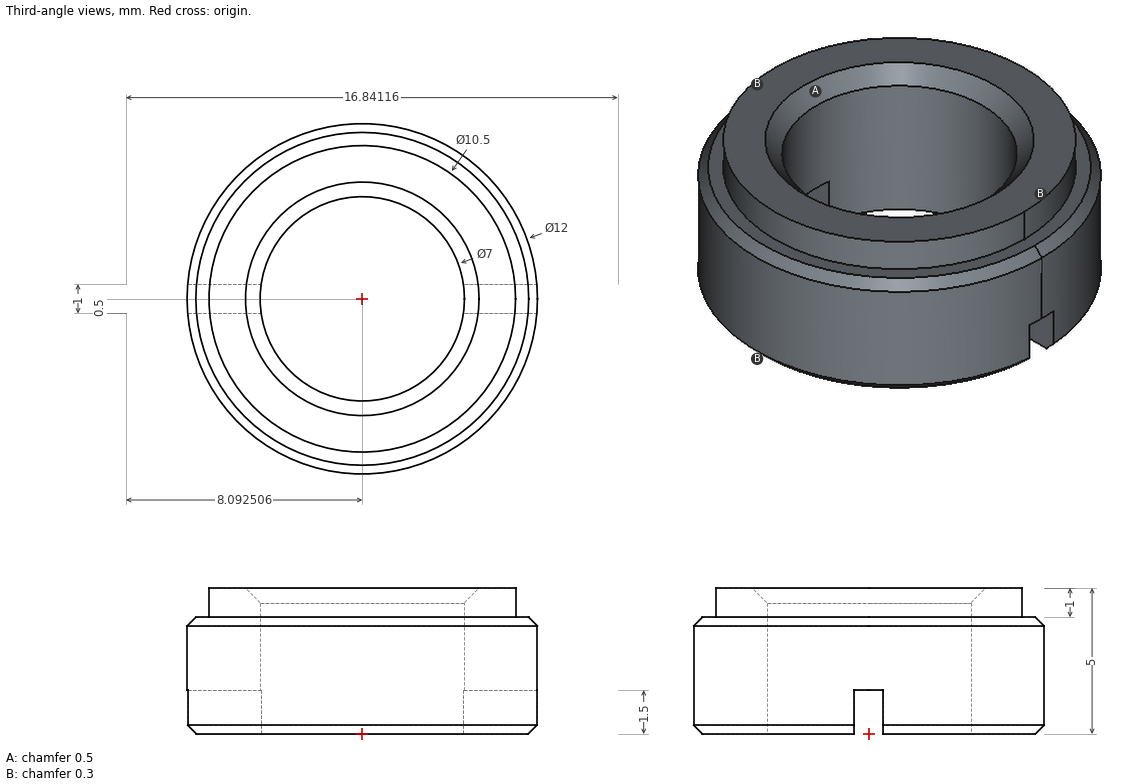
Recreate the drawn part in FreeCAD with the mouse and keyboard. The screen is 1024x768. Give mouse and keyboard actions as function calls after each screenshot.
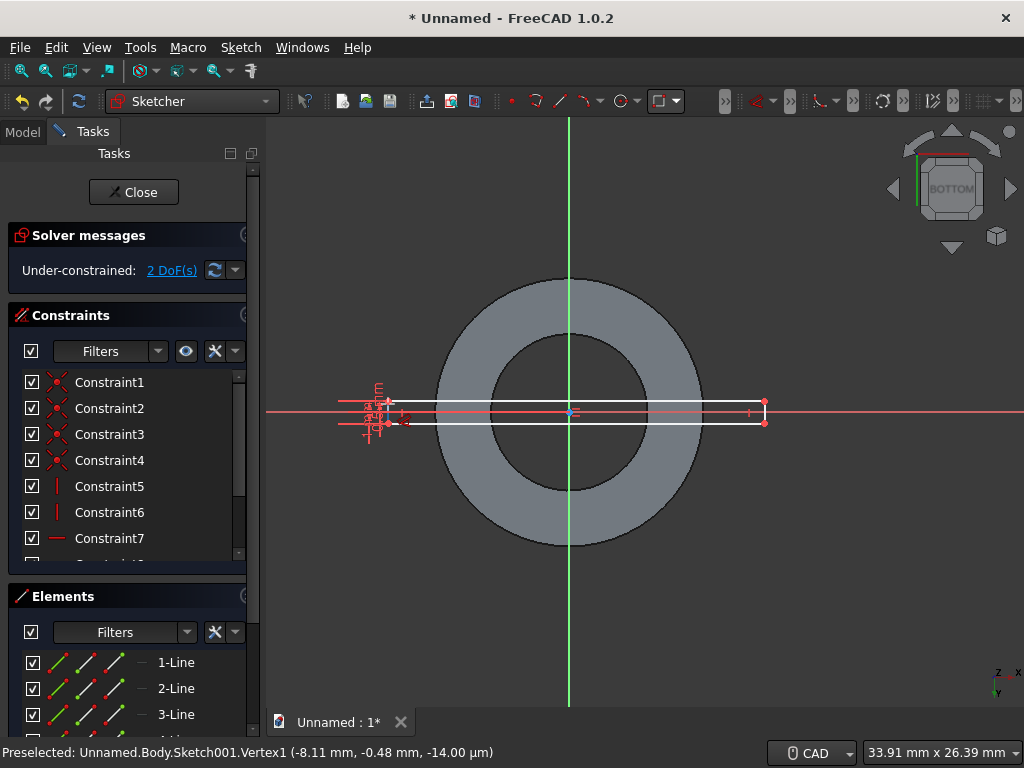
scroll(501, 424, up, 2)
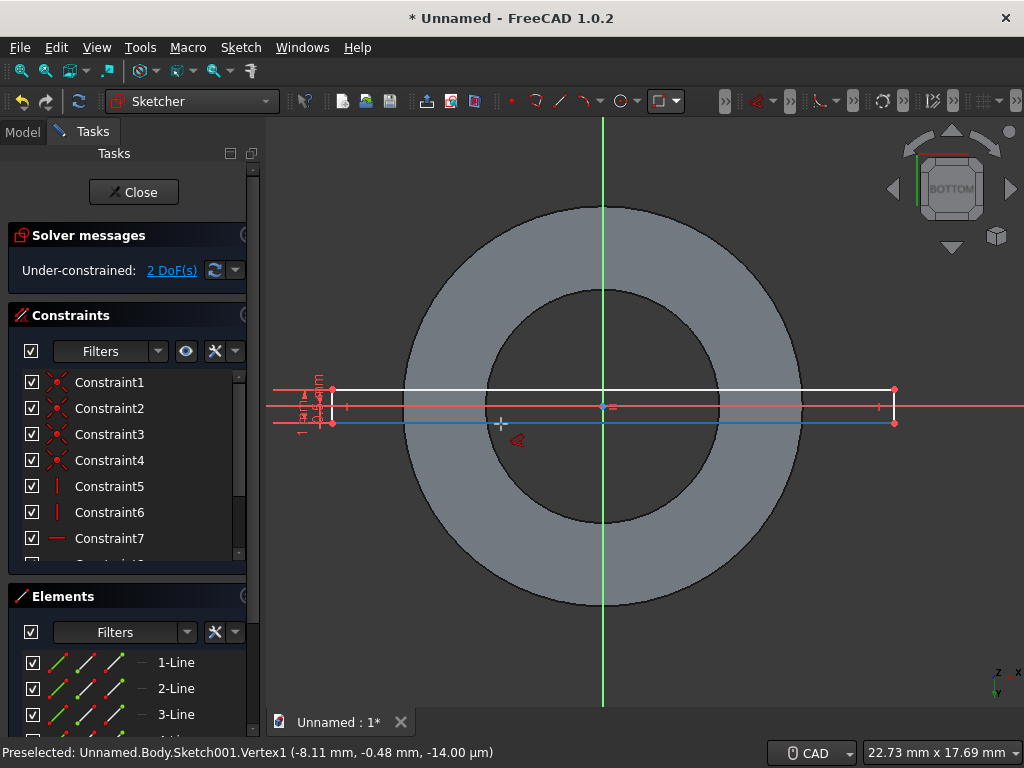
click(501, 423)
click(475, 457)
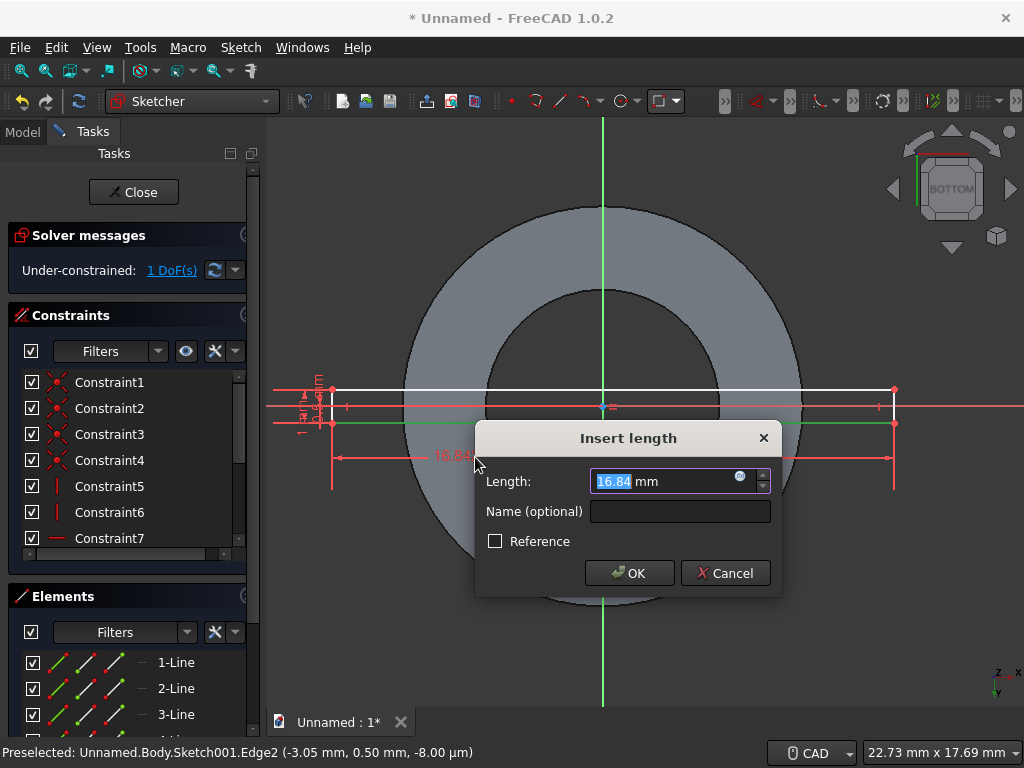
text(16.84116)
key(Return)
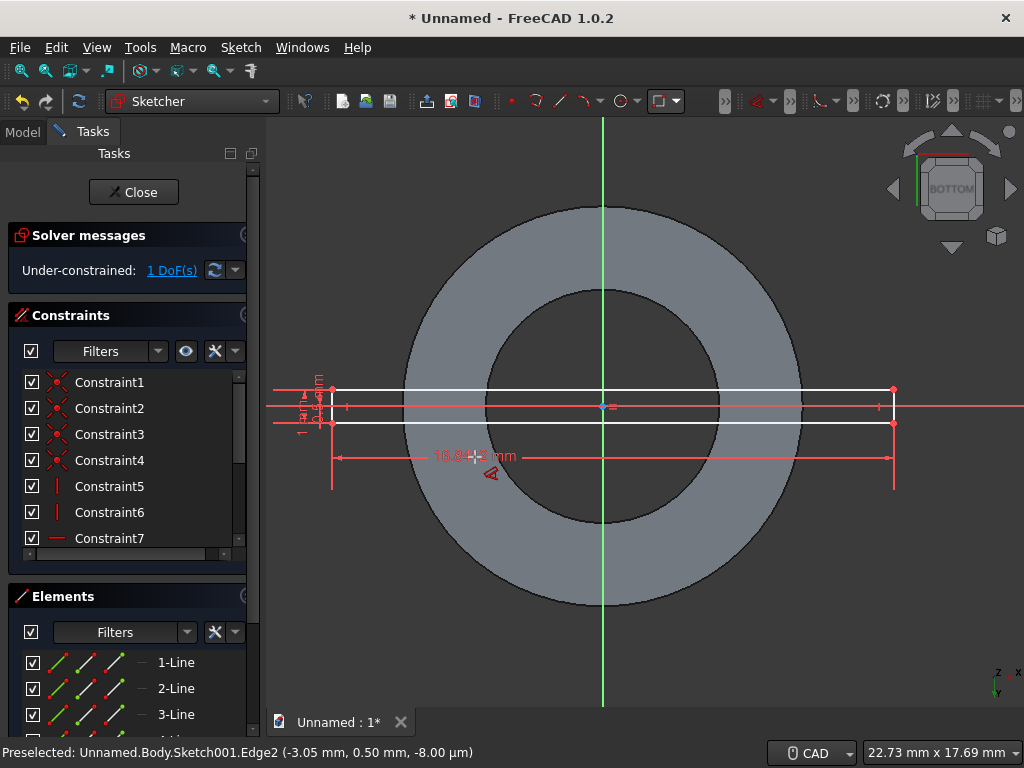
click(332, 390)
click(467, 356)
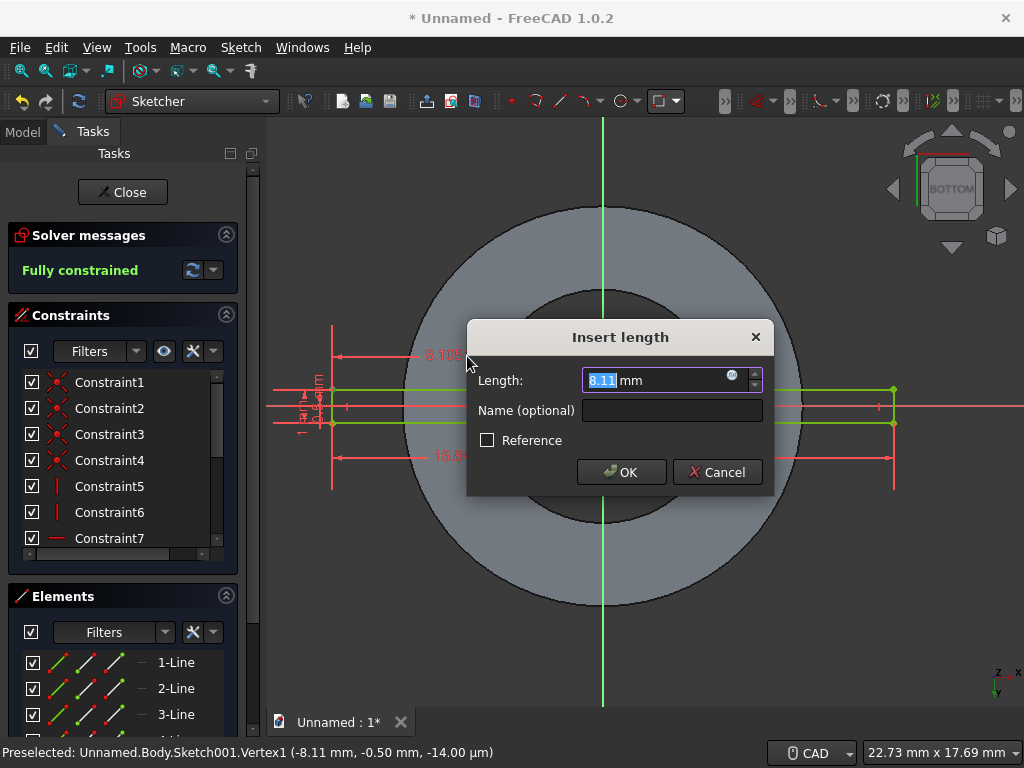
text(8.092506)
key(Return)
key(Escape)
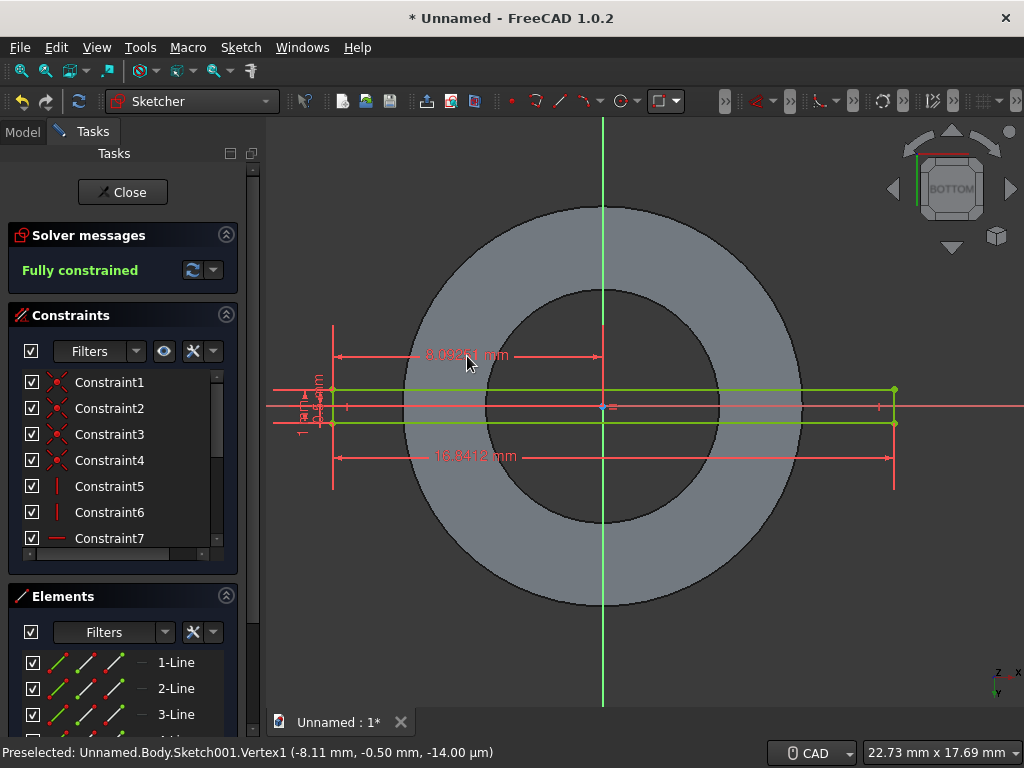
click(123, 192)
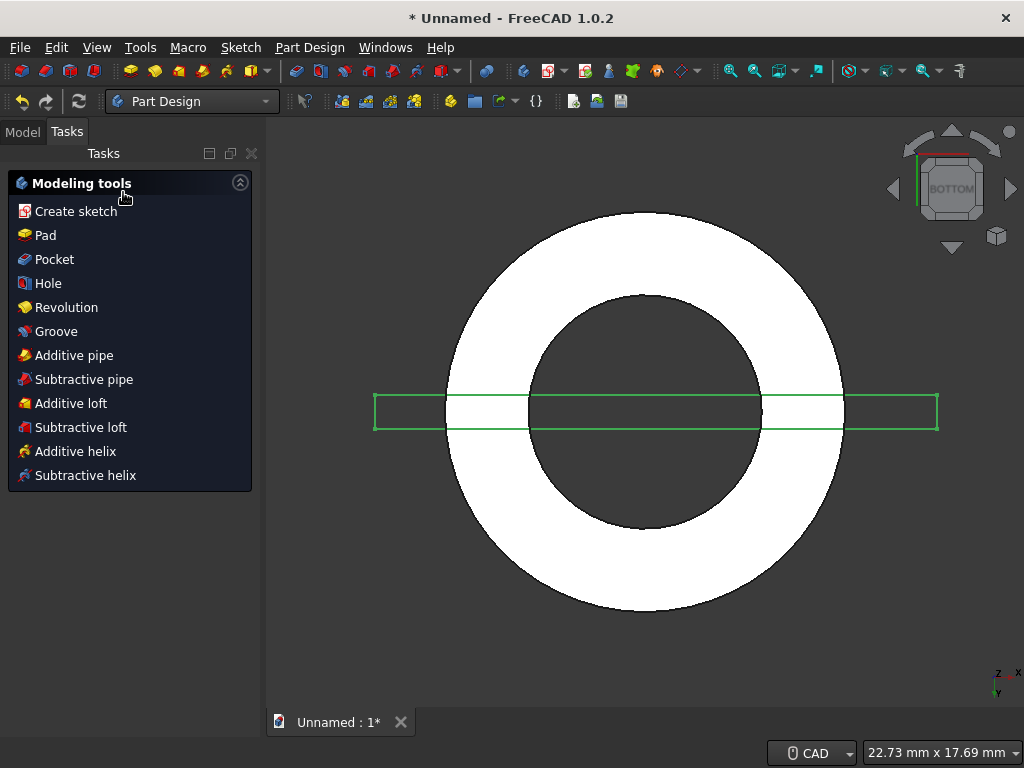
click(298, 72)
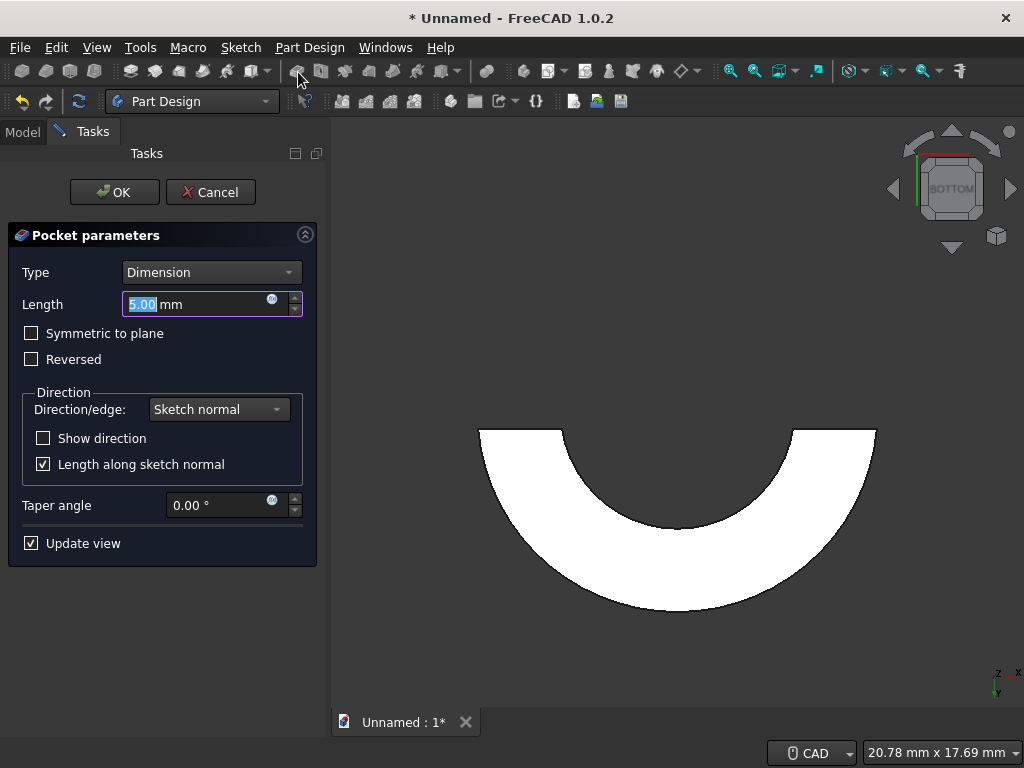
text(1.5)
key(Tab)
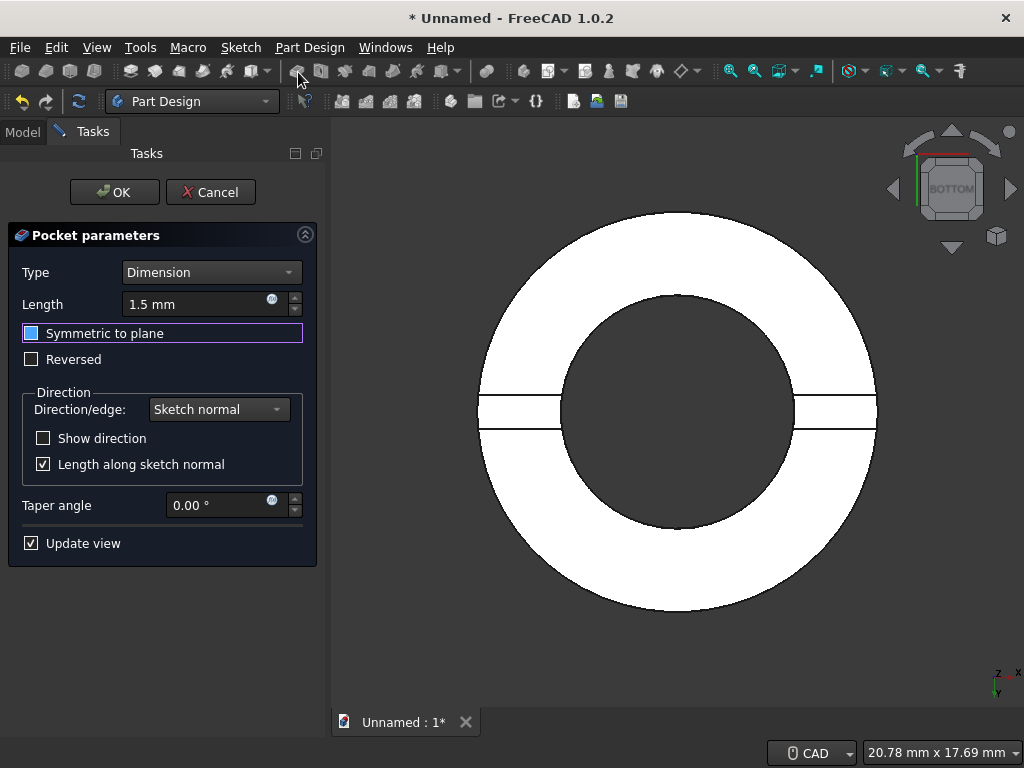
click(115, 192)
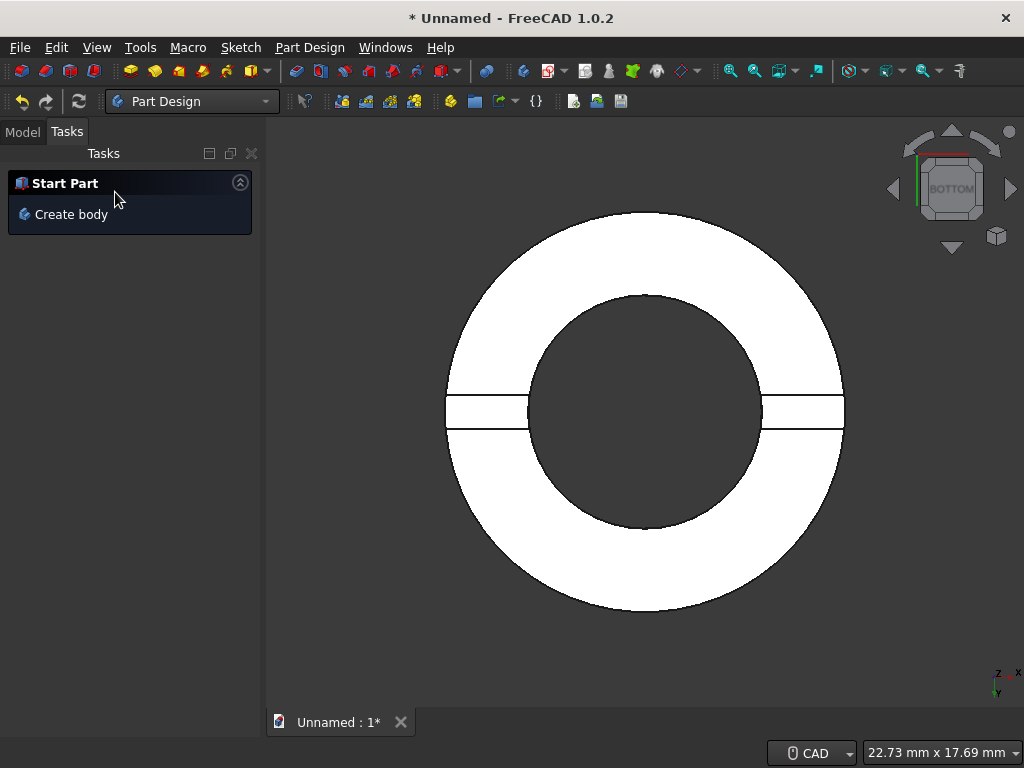
click(23, 131)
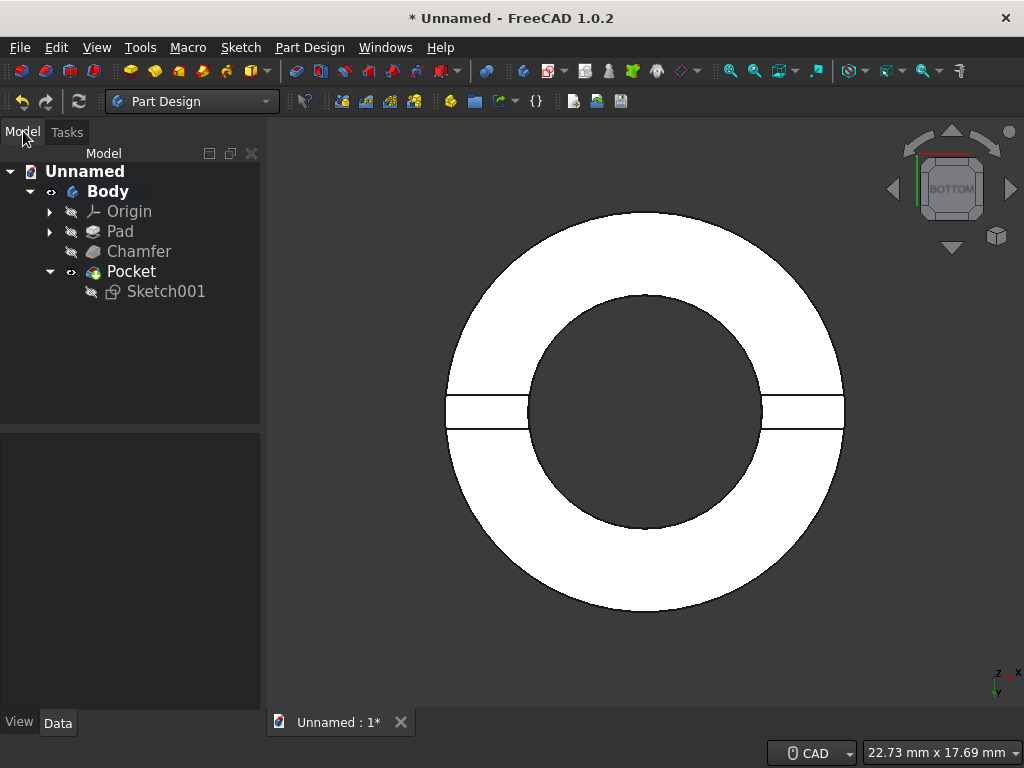
click(50, 212)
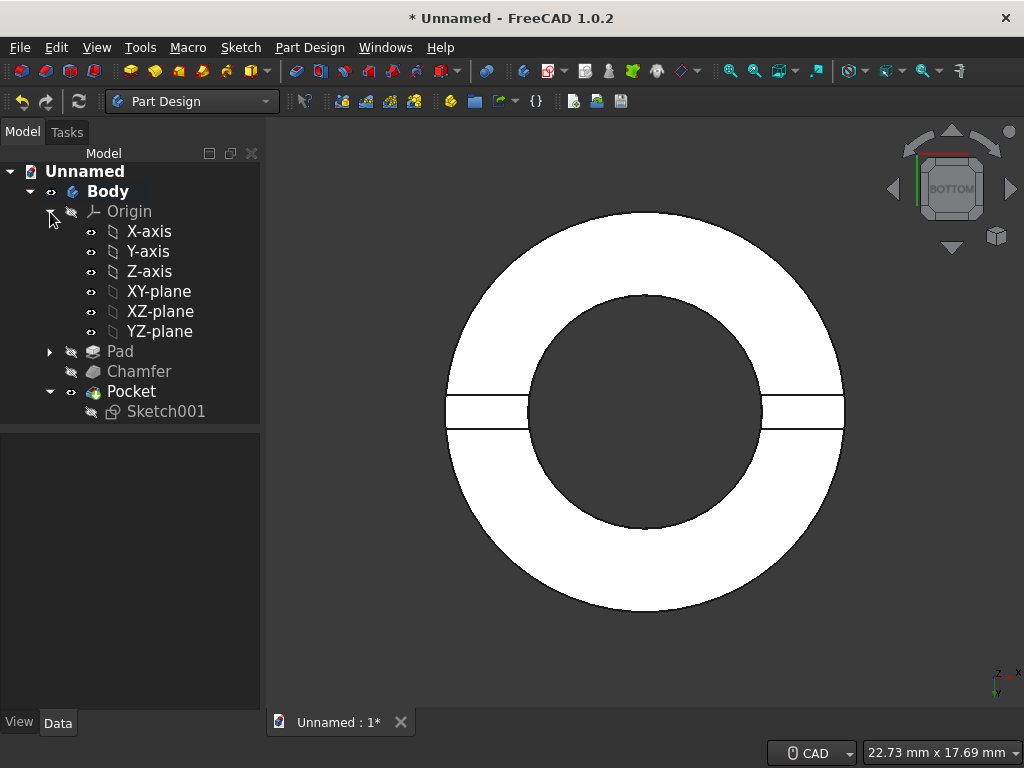
click(136, 292)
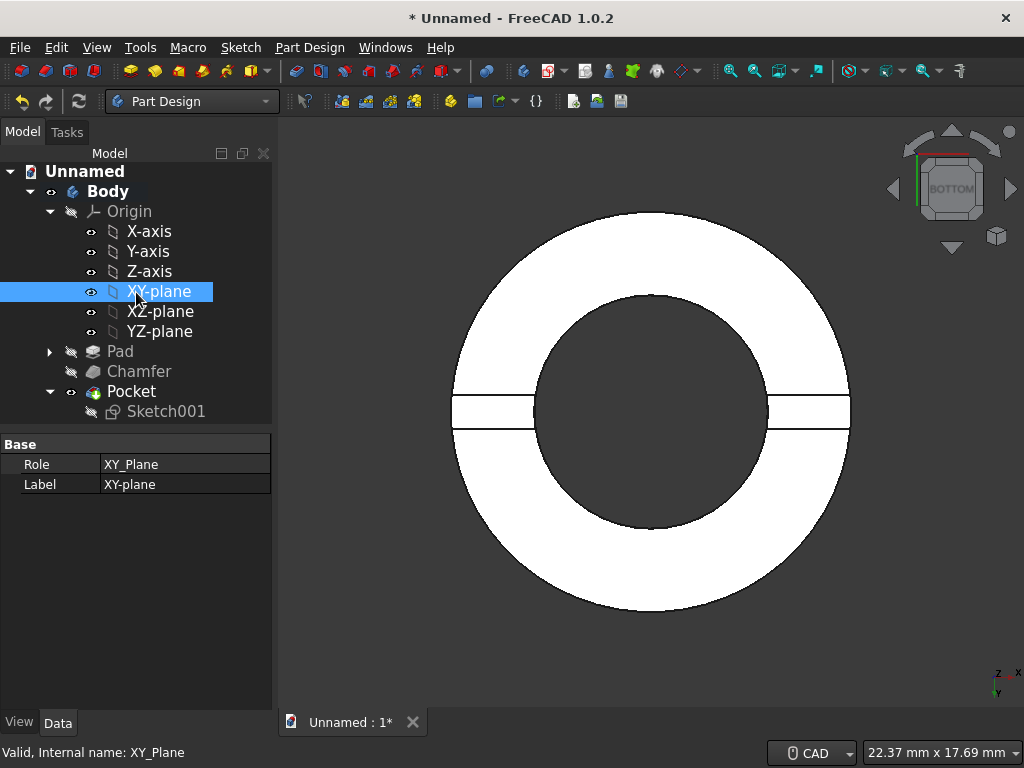
click(682, 72)